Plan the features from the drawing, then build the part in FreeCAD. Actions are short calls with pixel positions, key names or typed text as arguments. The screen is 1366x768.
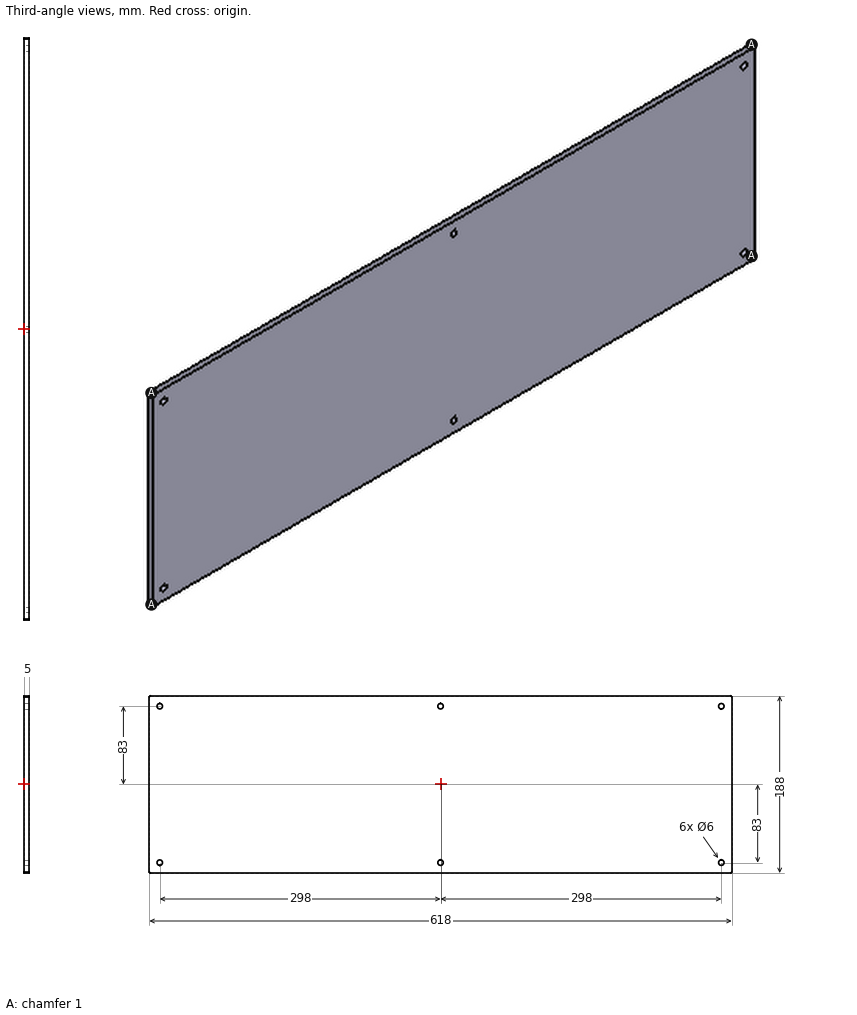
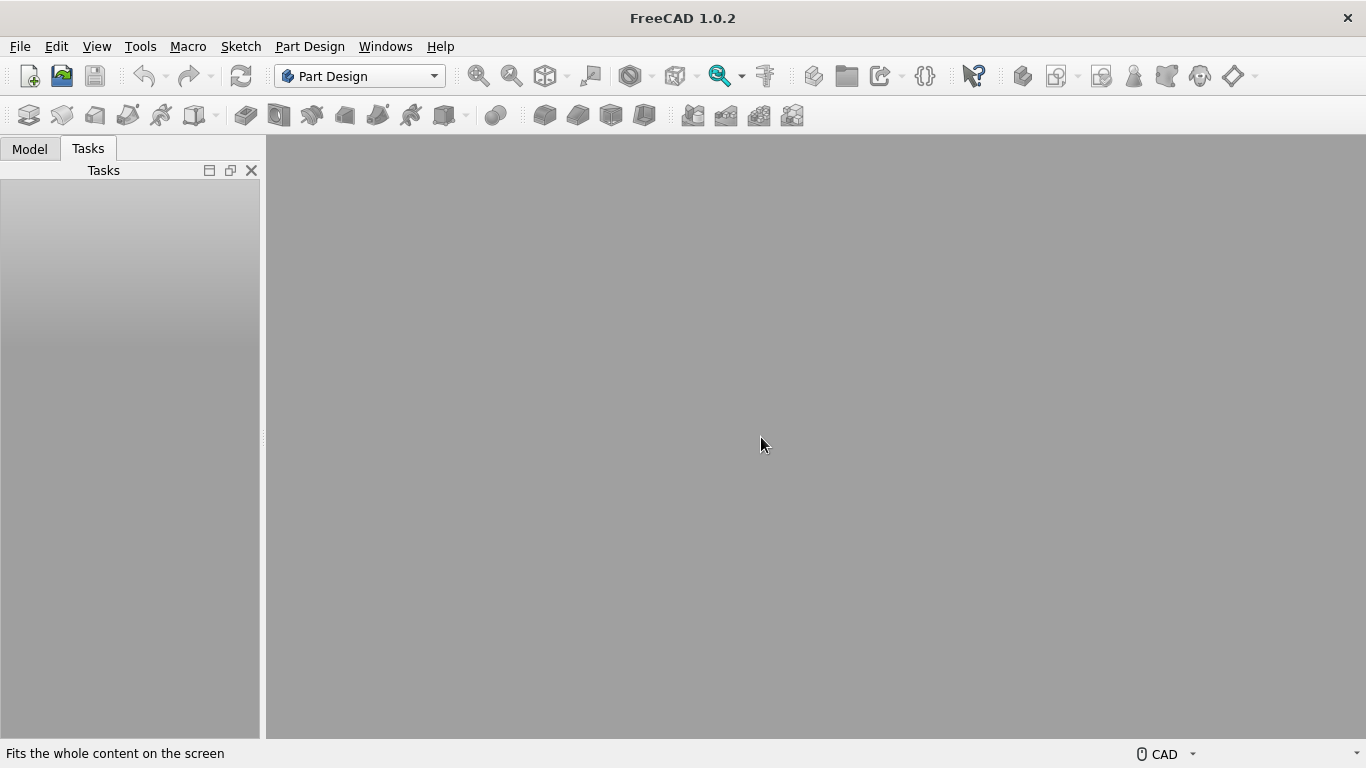
click(29, 76)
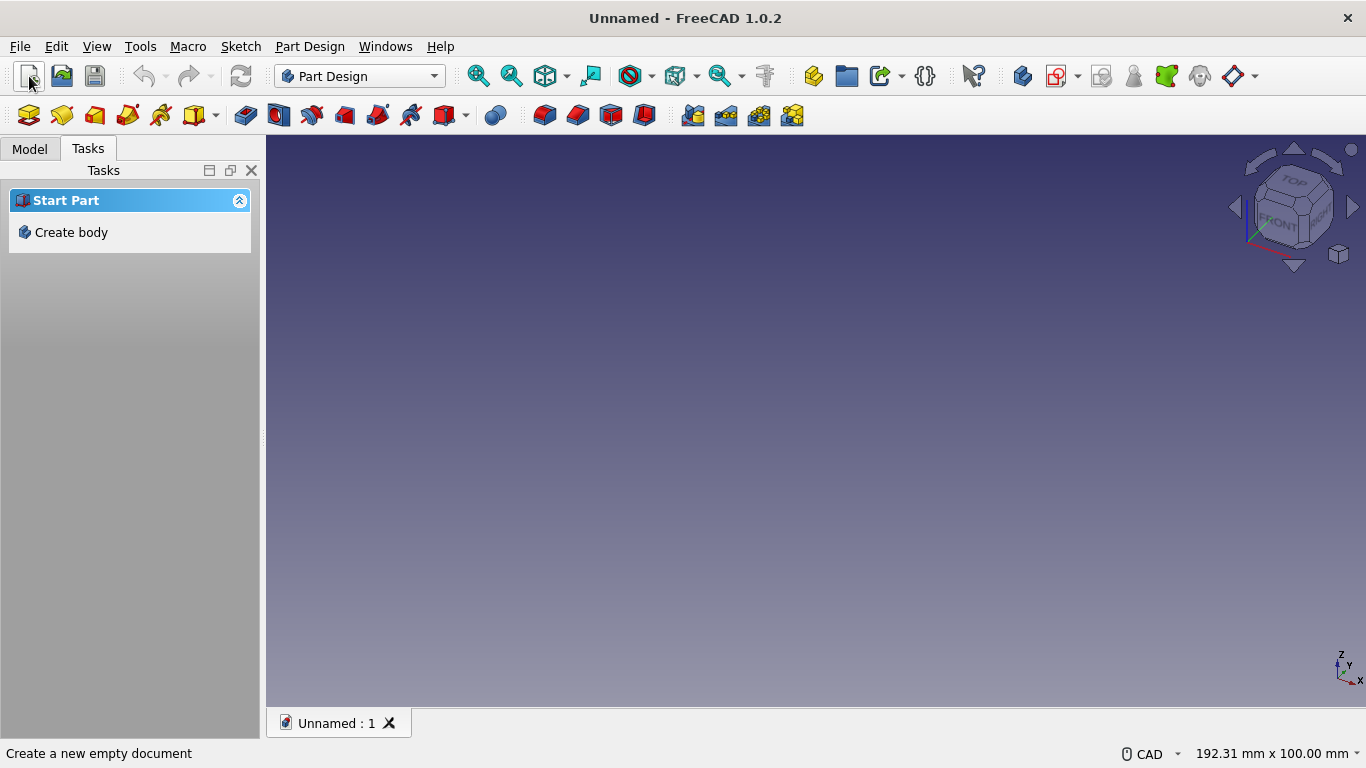
click(1056, 76)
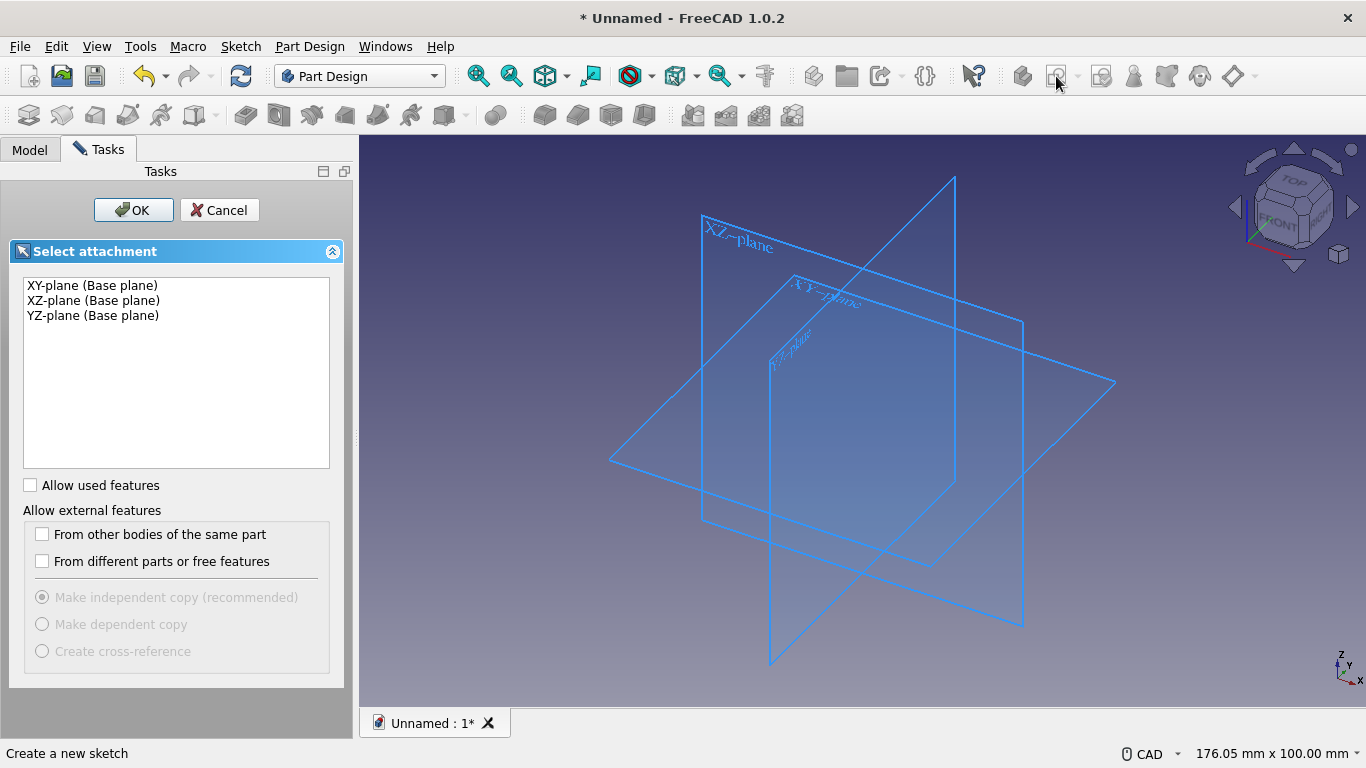
click(84, 316)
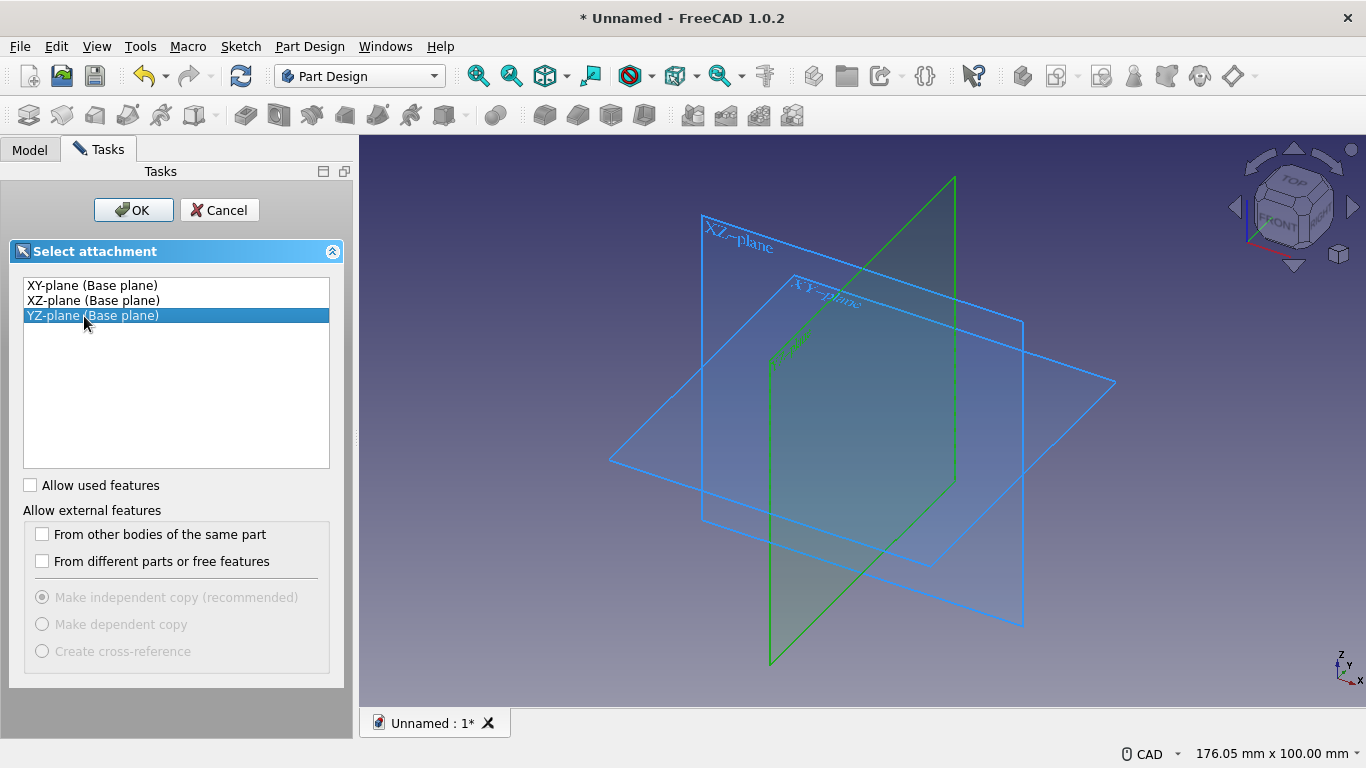
click(134, 210)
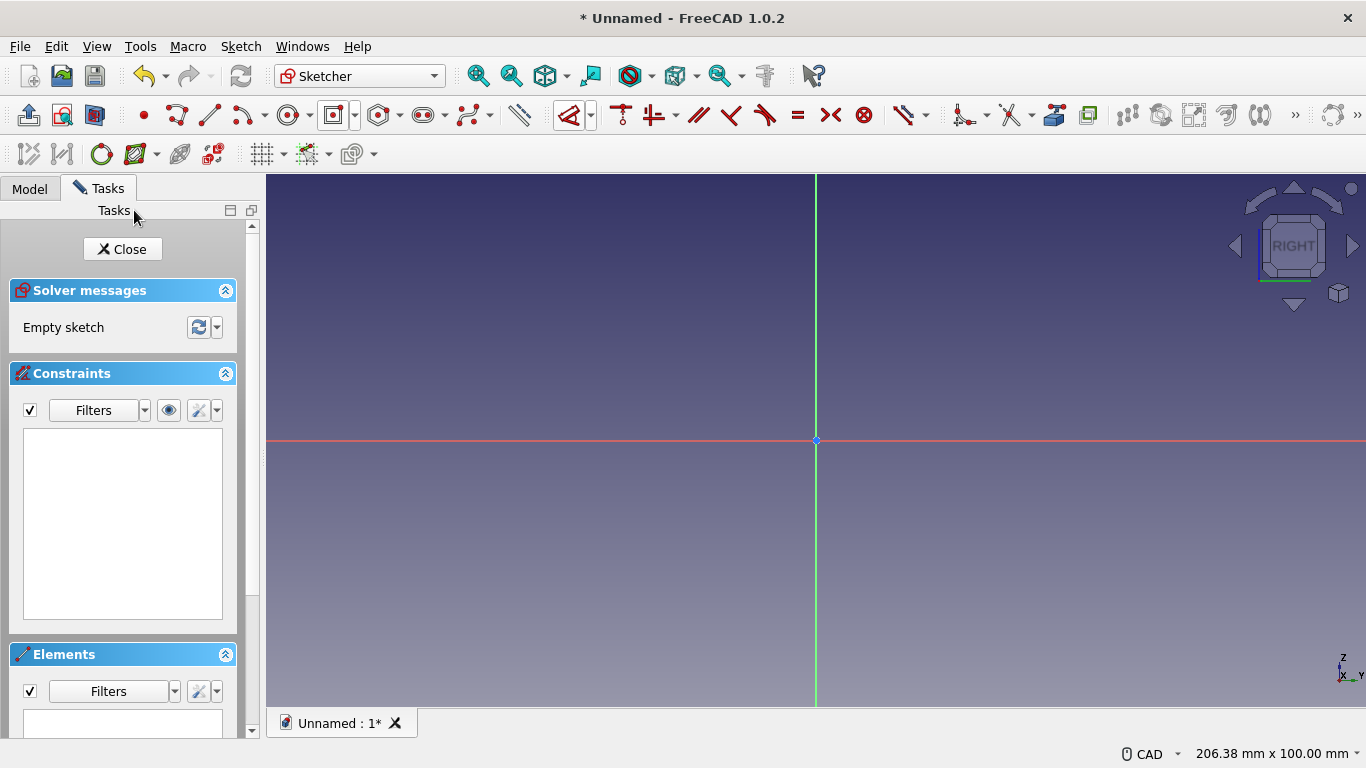
scroll(730, 440, down, 8)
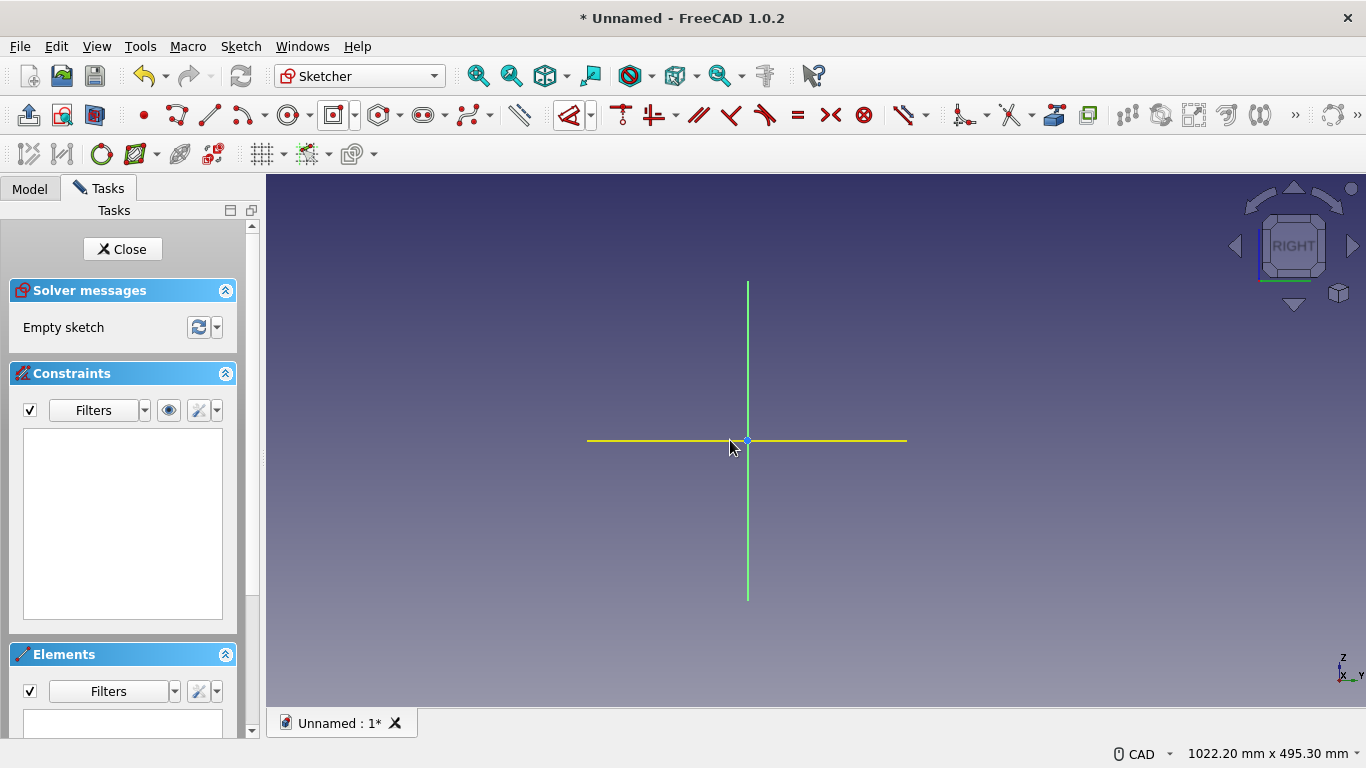
click(332, 116)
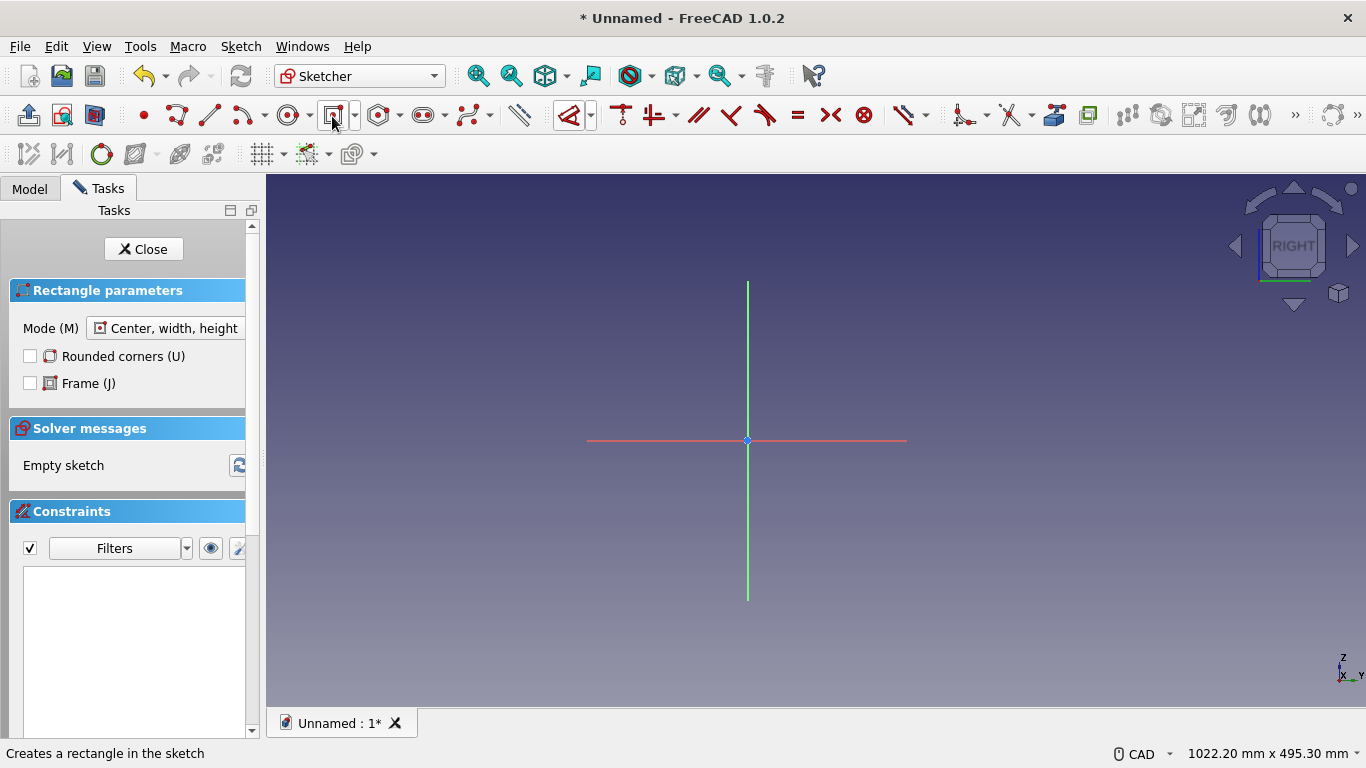
click(748, 440)
click(1080, 339)
key(Escape)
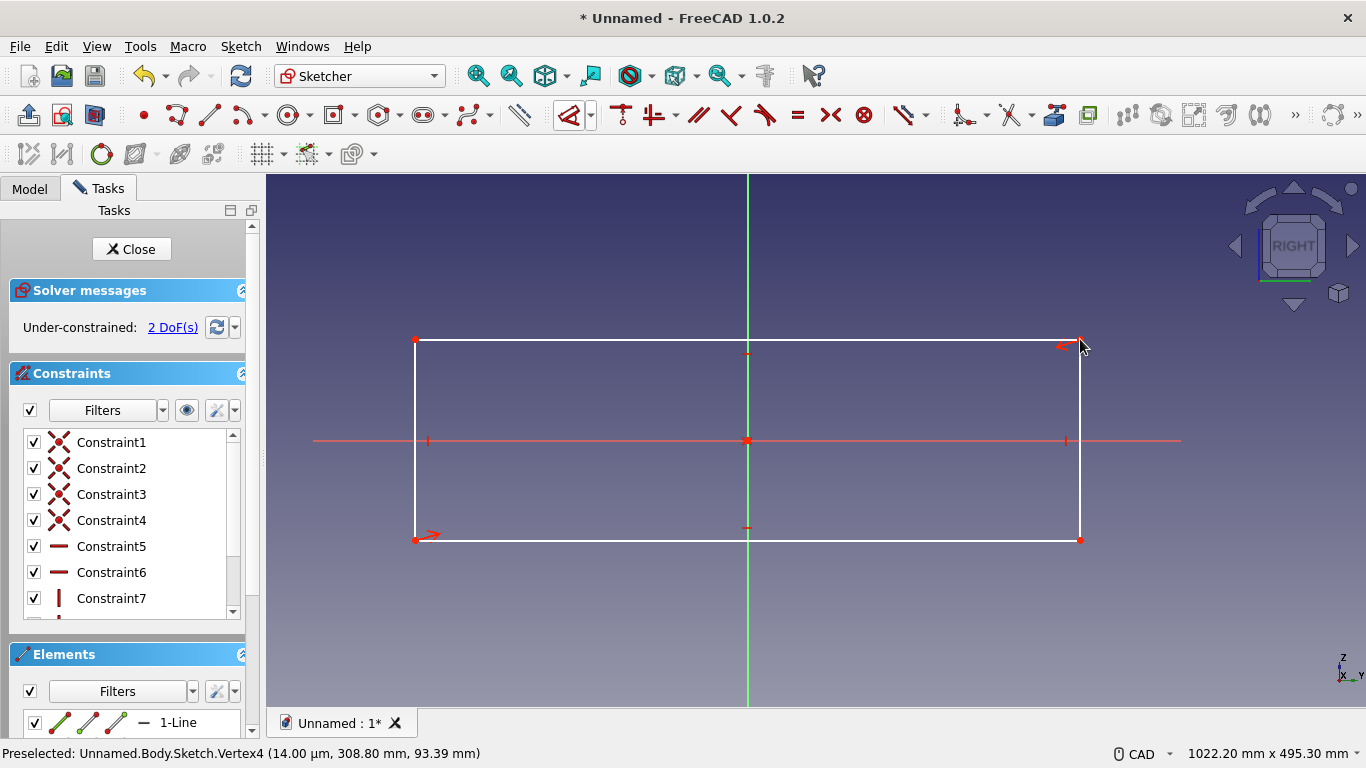
click(568, 116)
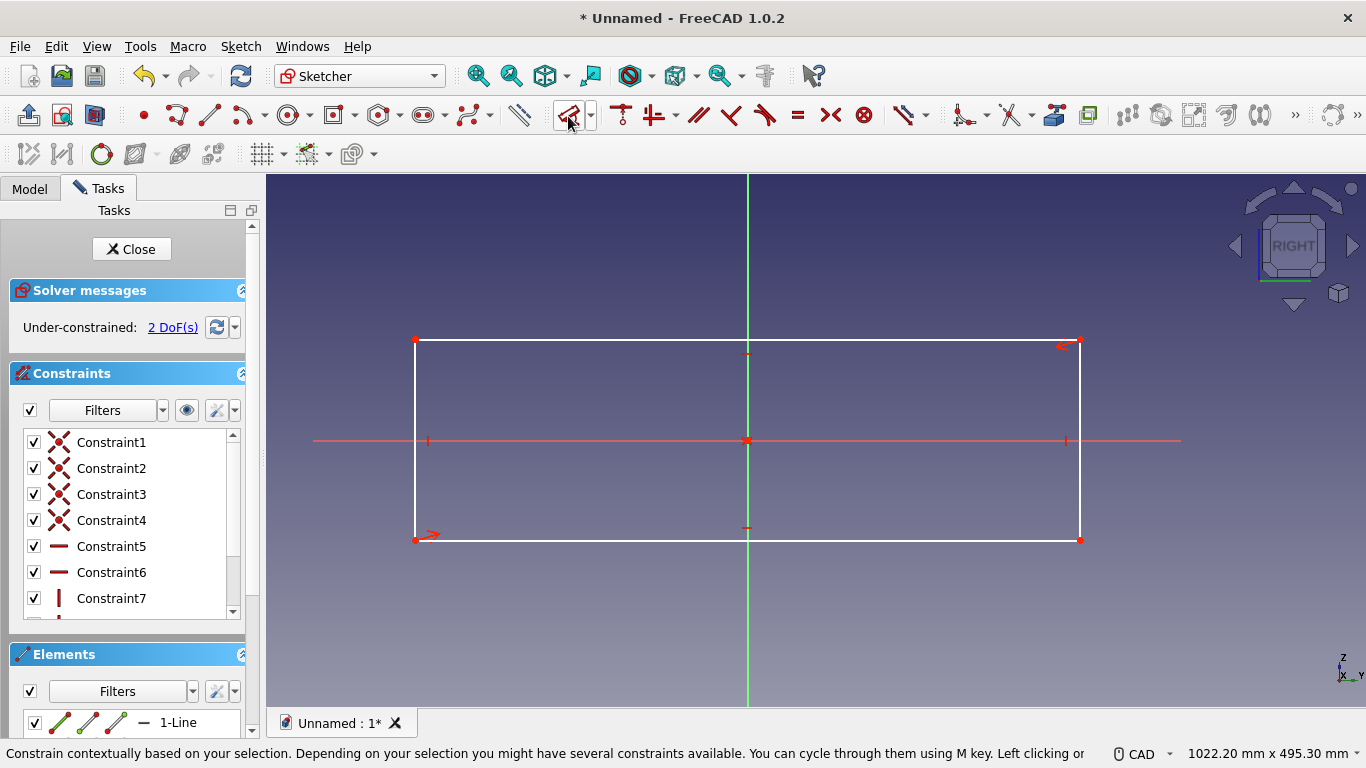
click(615, 541)
click(595, 575)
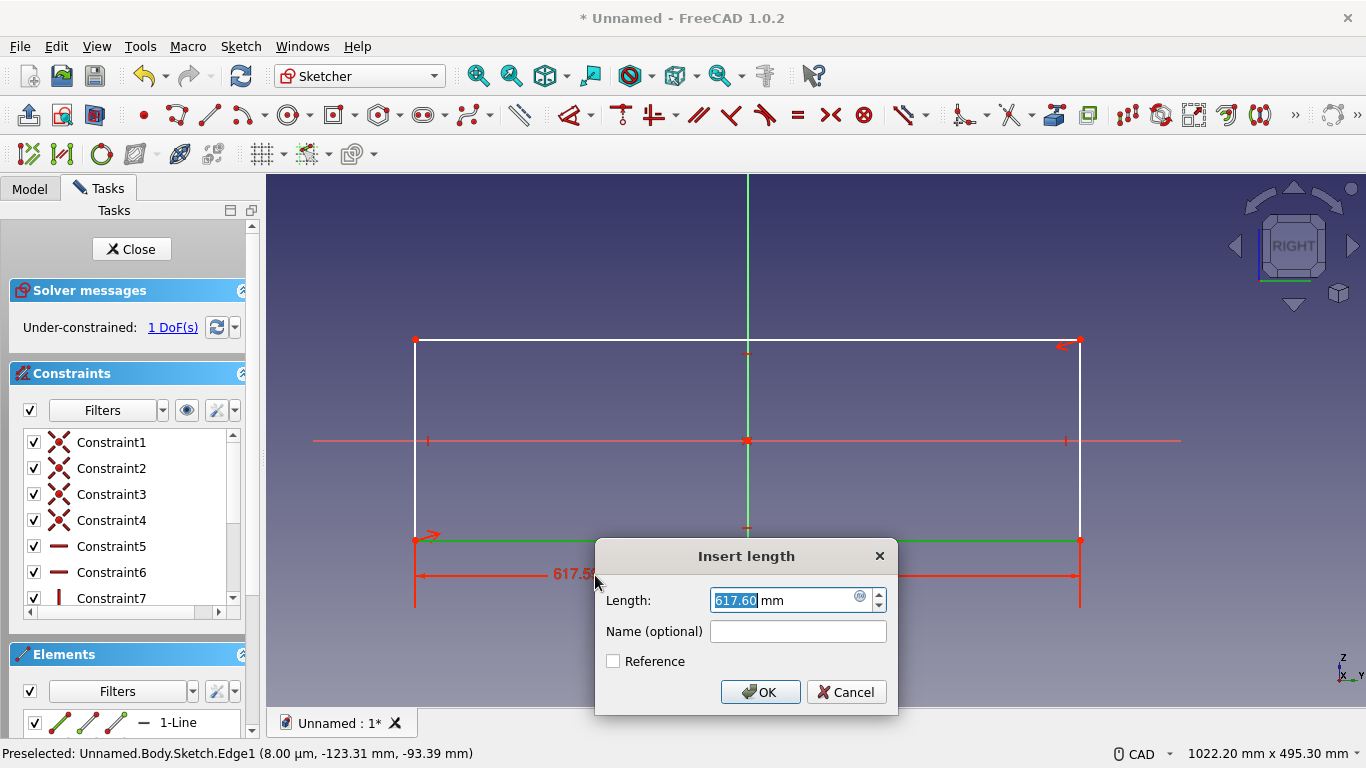
text(618)
key(Return)